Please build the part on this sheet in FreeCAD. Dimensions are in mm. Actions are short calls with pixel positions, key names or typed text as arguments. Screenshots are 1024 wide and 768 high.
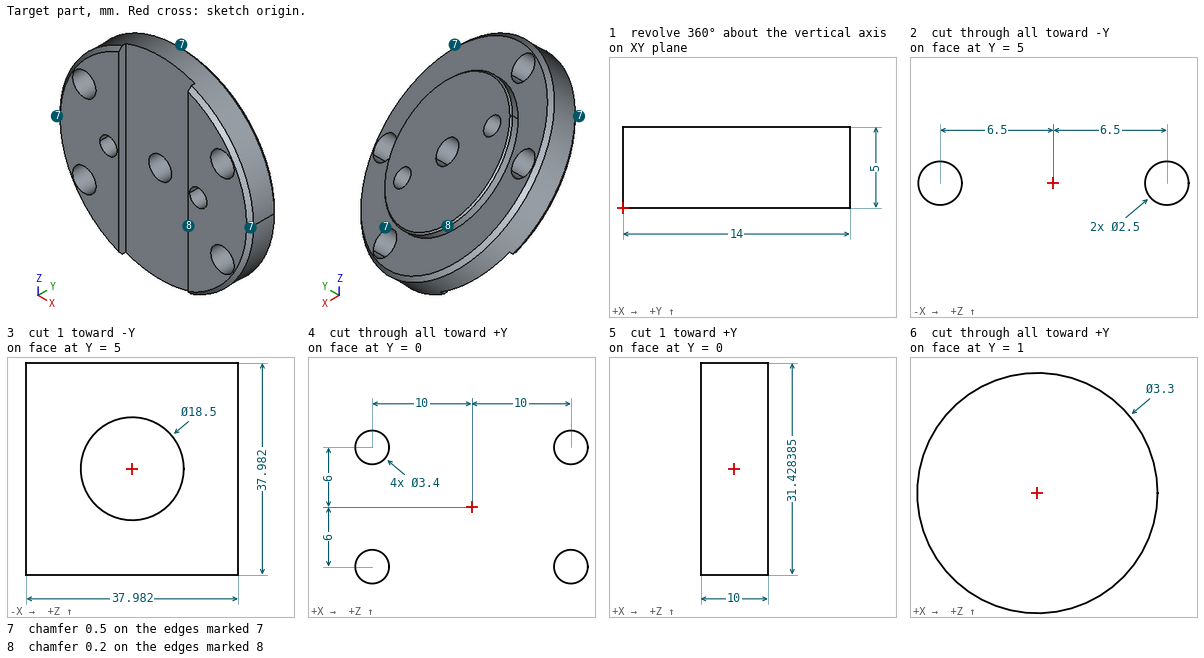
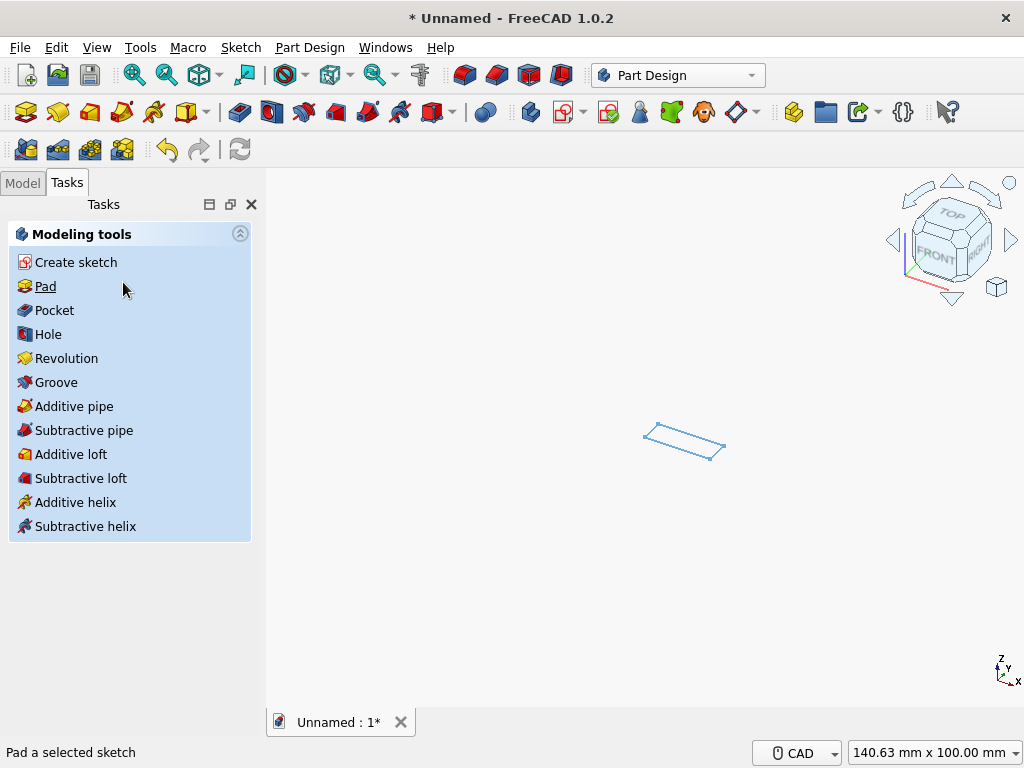
click(58, 112)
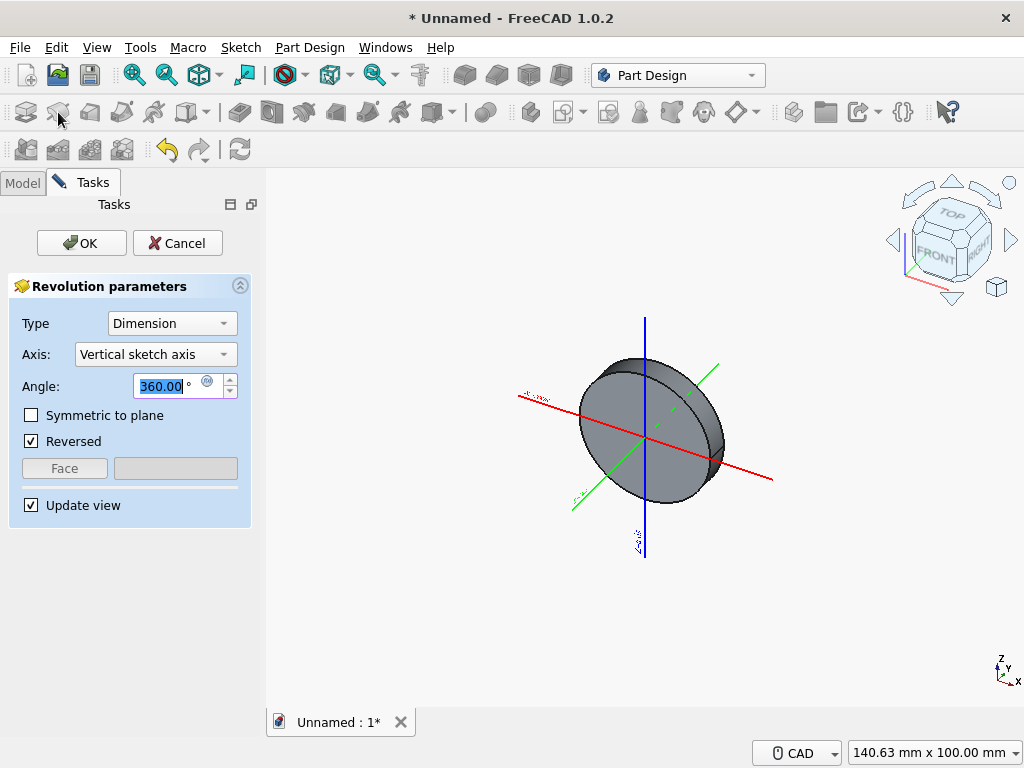
click(82, 243)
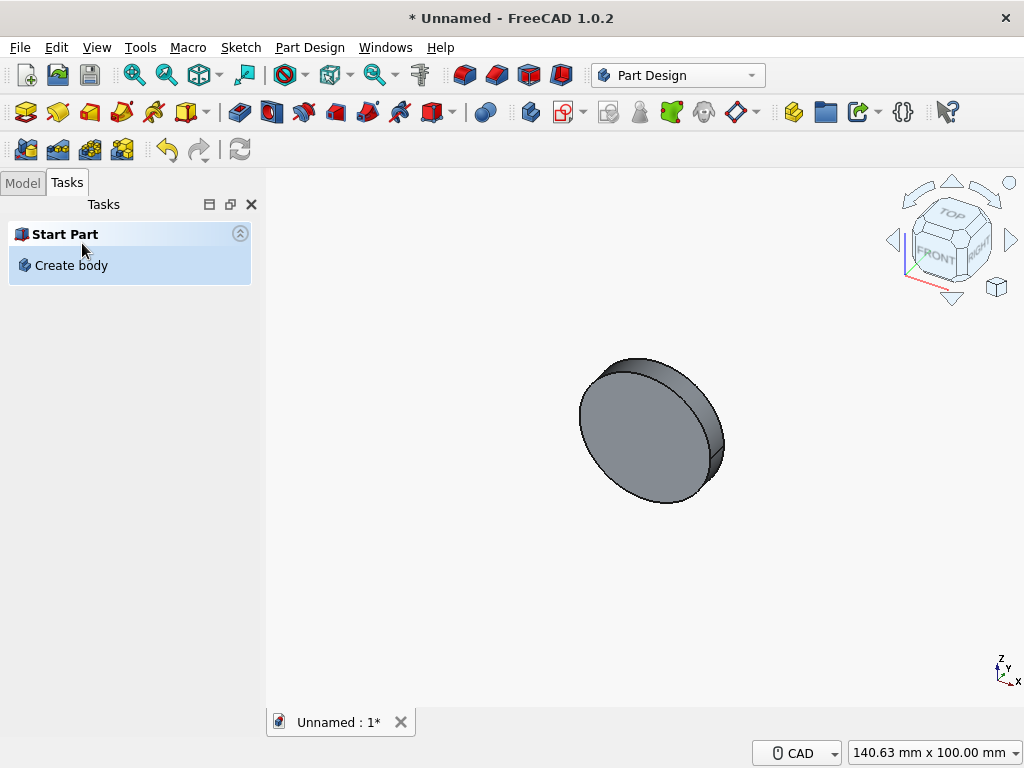
key(v)
key(f)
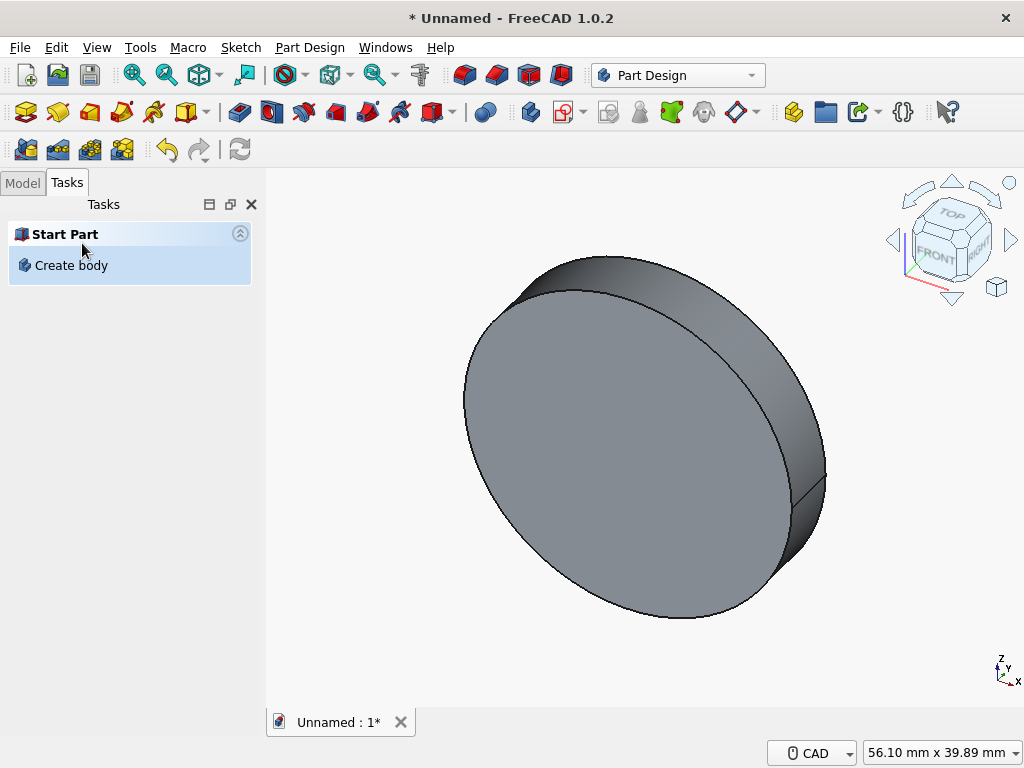
key(4)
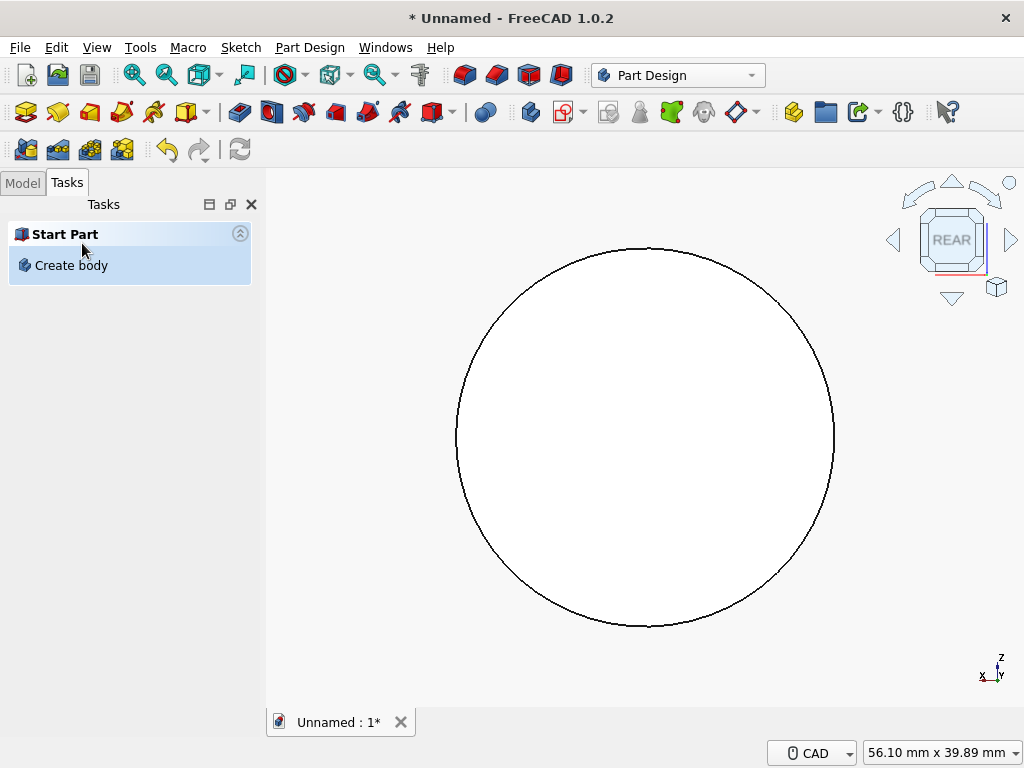
click(645, 436)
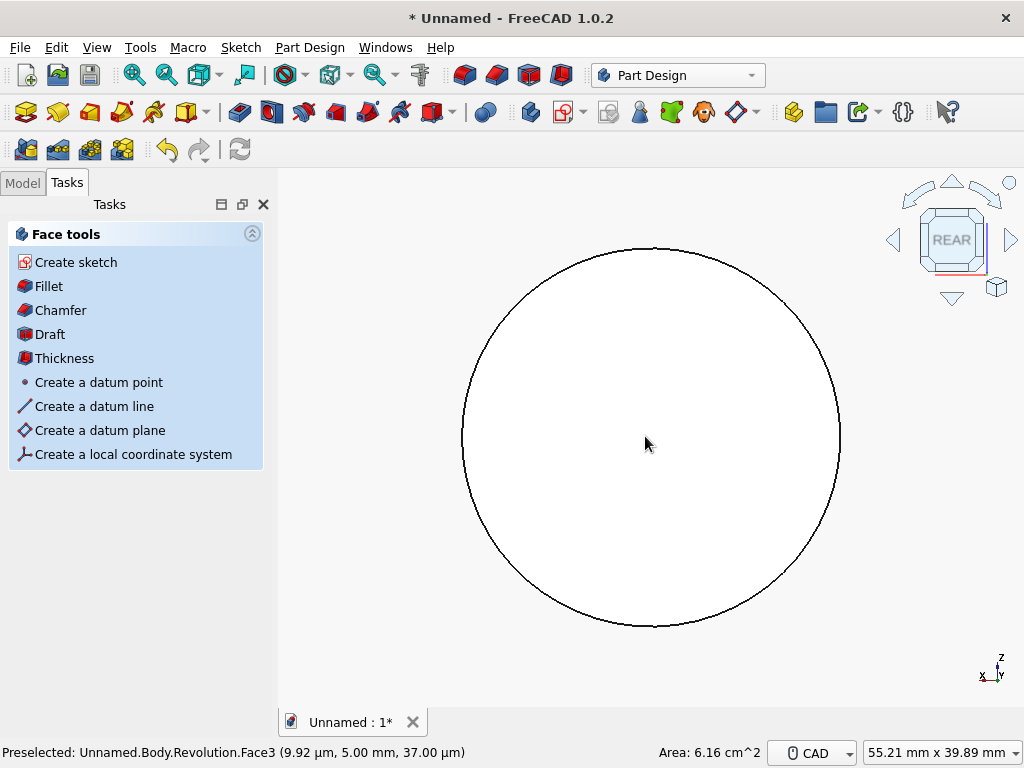
click(564, 112)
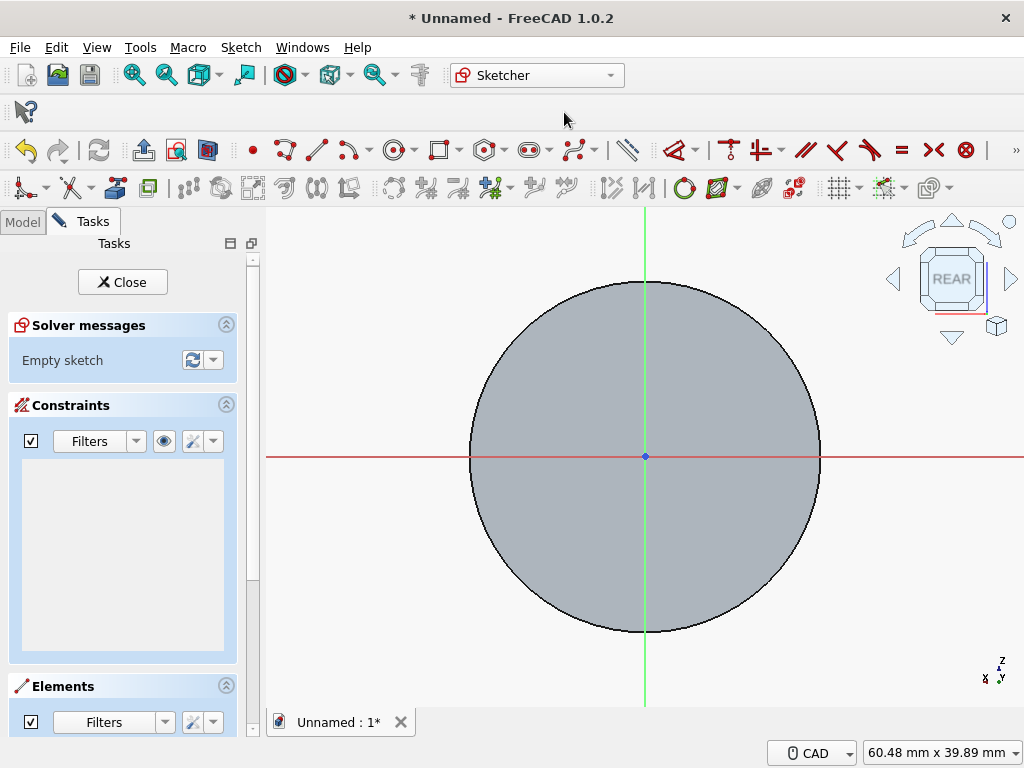
scroll(701, 457, up, 4)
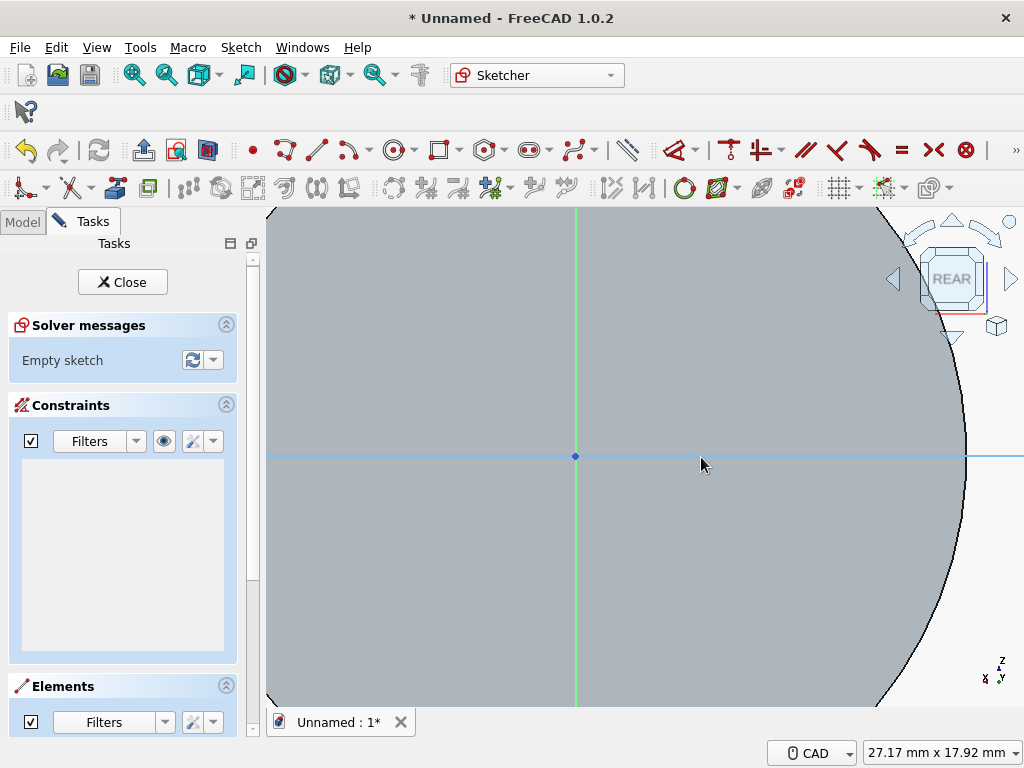
key(g)
key(c)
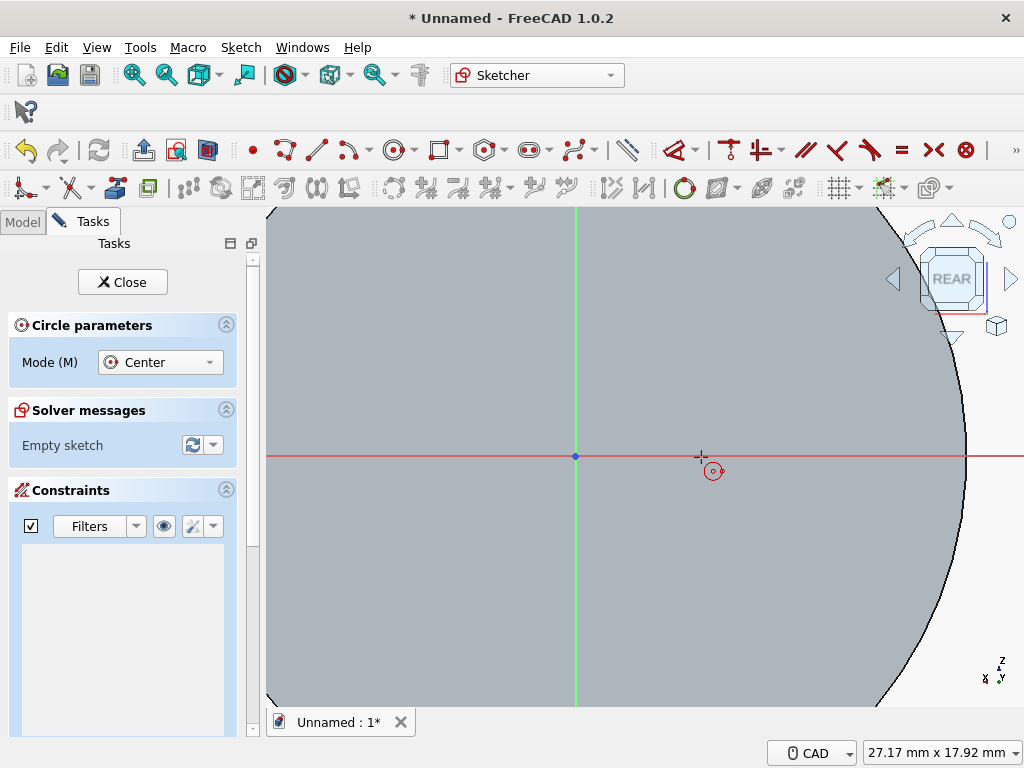
click(757, 456)
click(782, 432)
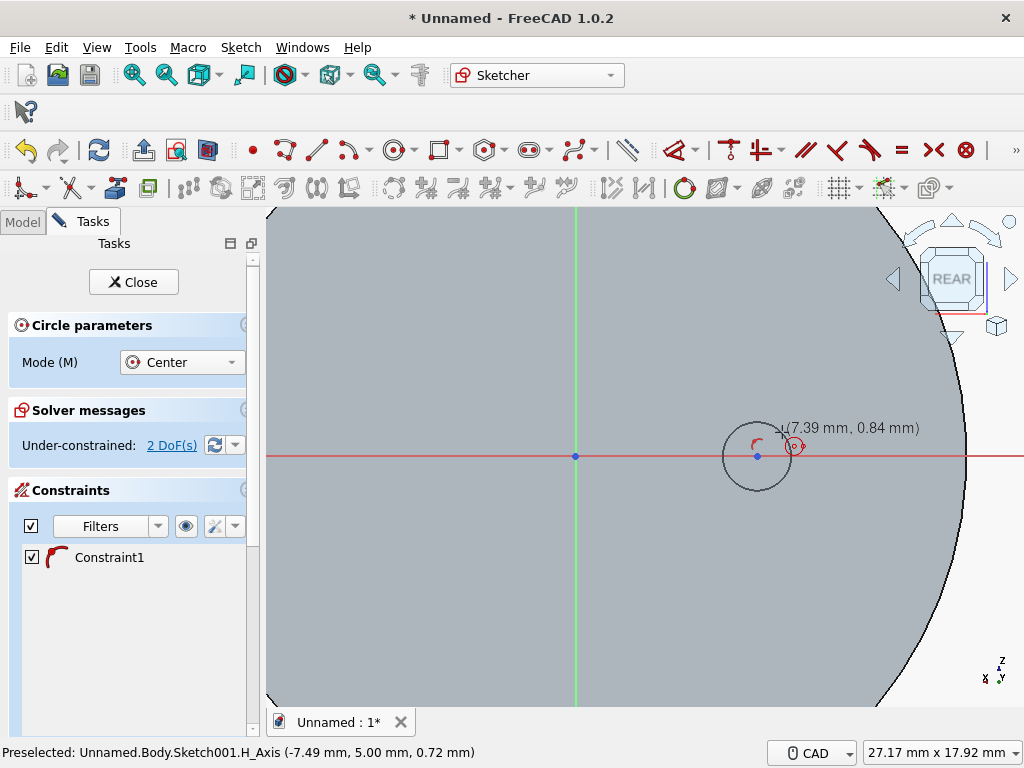
click(395, 456)
click(419, 432)
key(Escape)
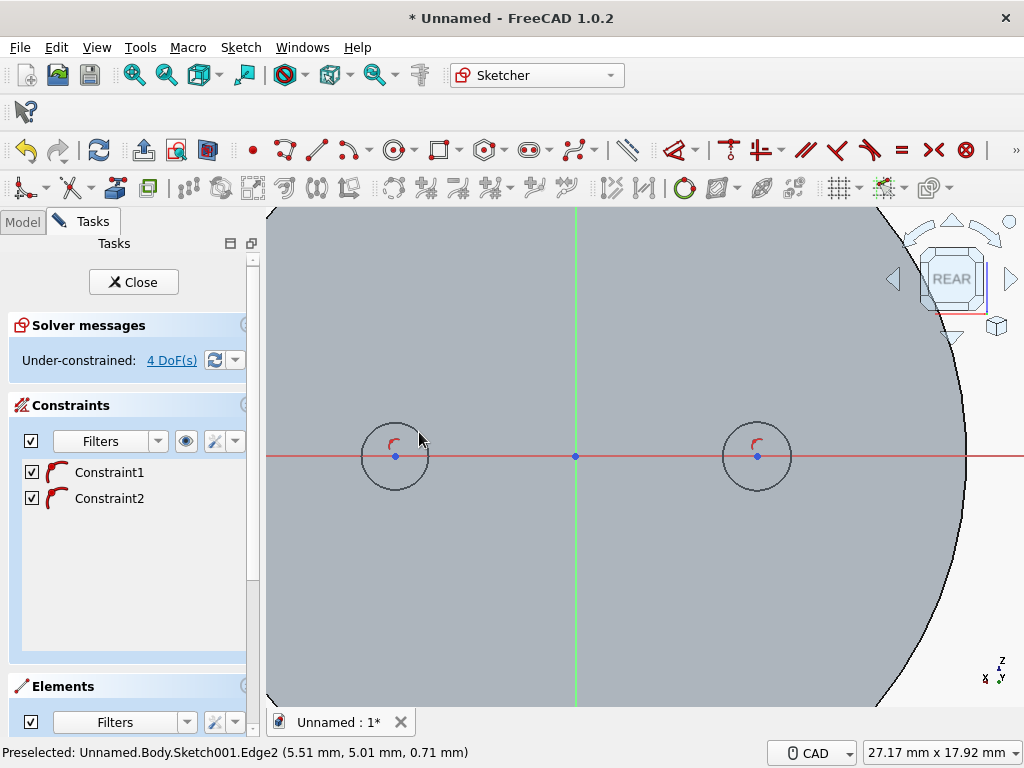
click(781, 432)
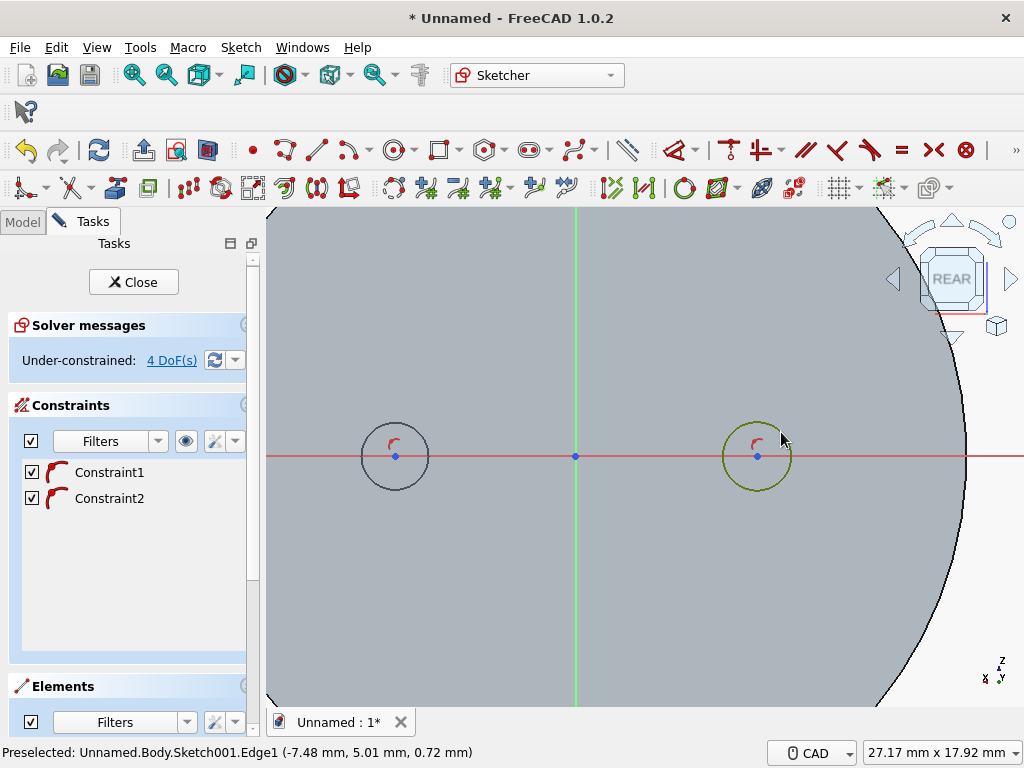
click(419, 433)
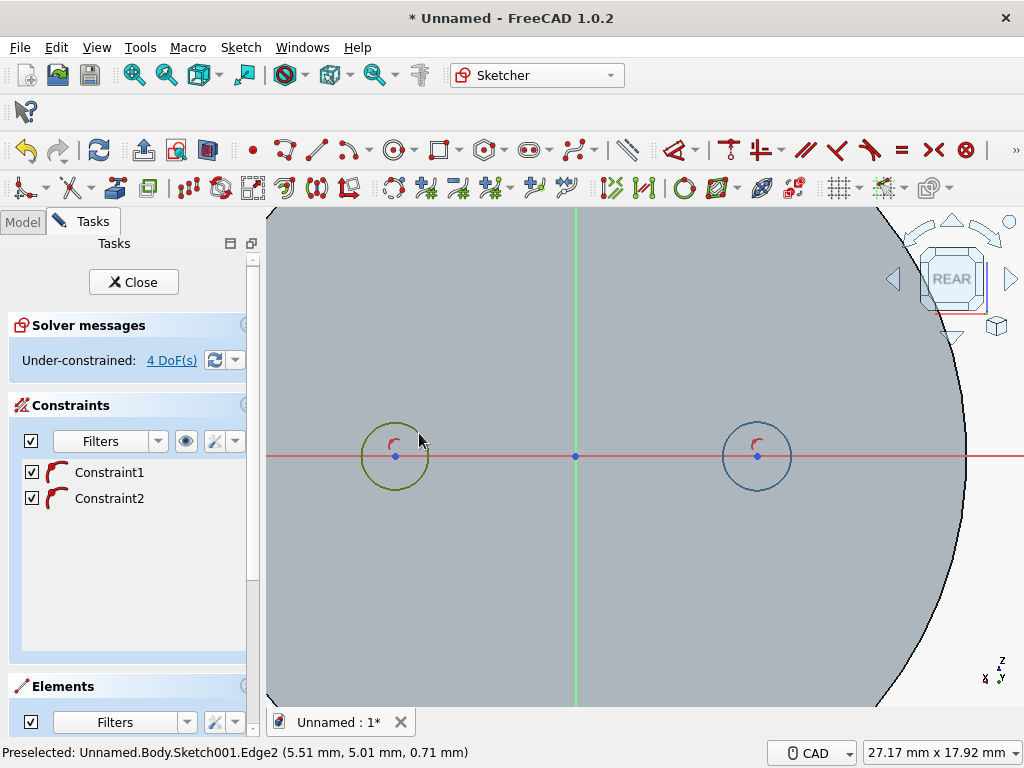
key(e)